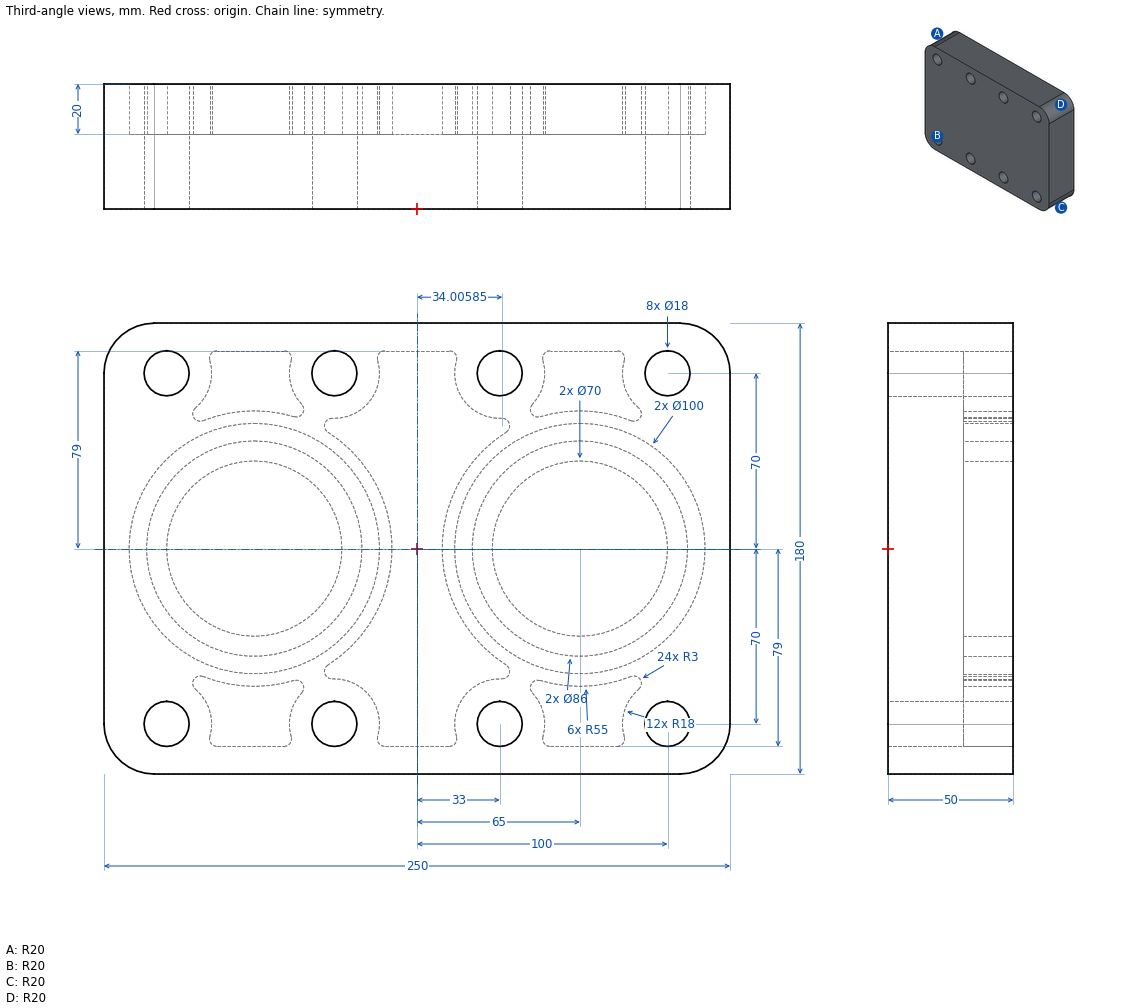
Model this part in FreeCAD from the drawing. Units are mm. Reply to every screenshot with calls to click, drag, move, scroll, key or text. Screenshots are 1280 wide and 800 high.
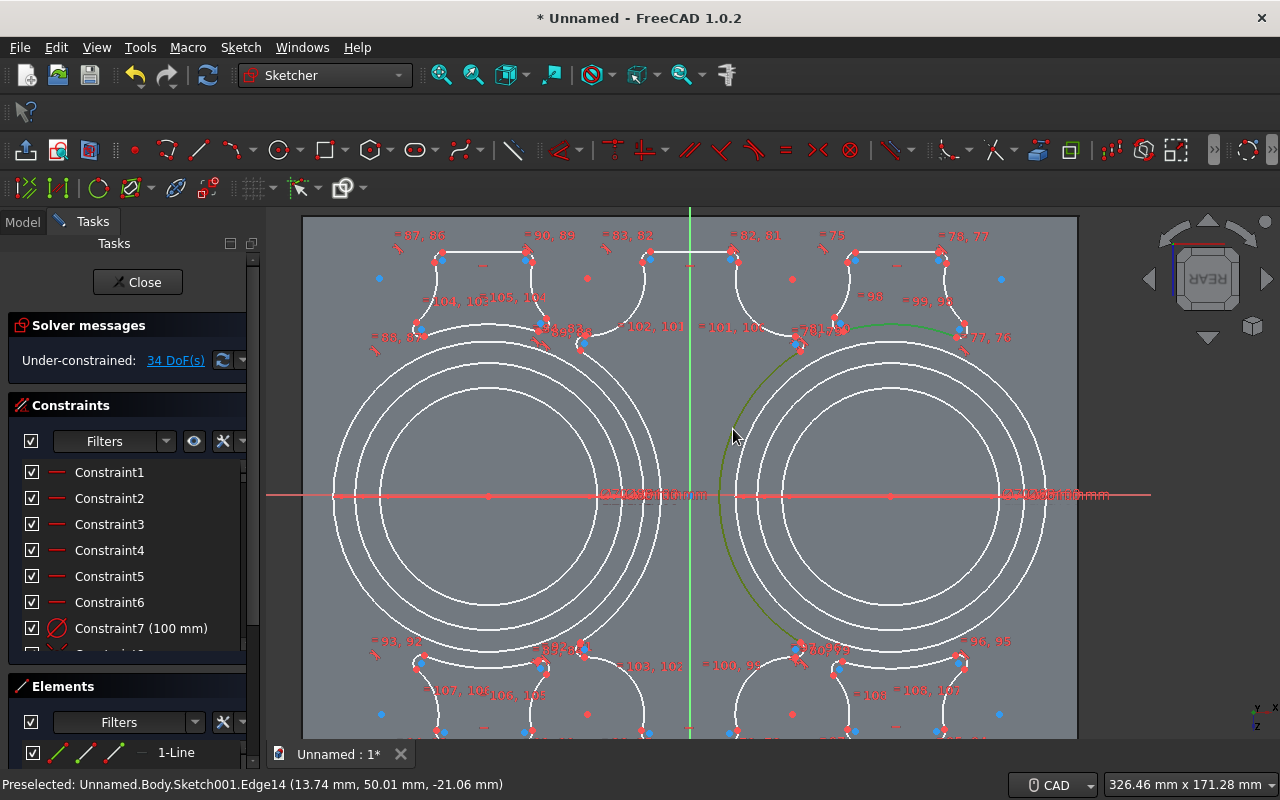
click(647, 564)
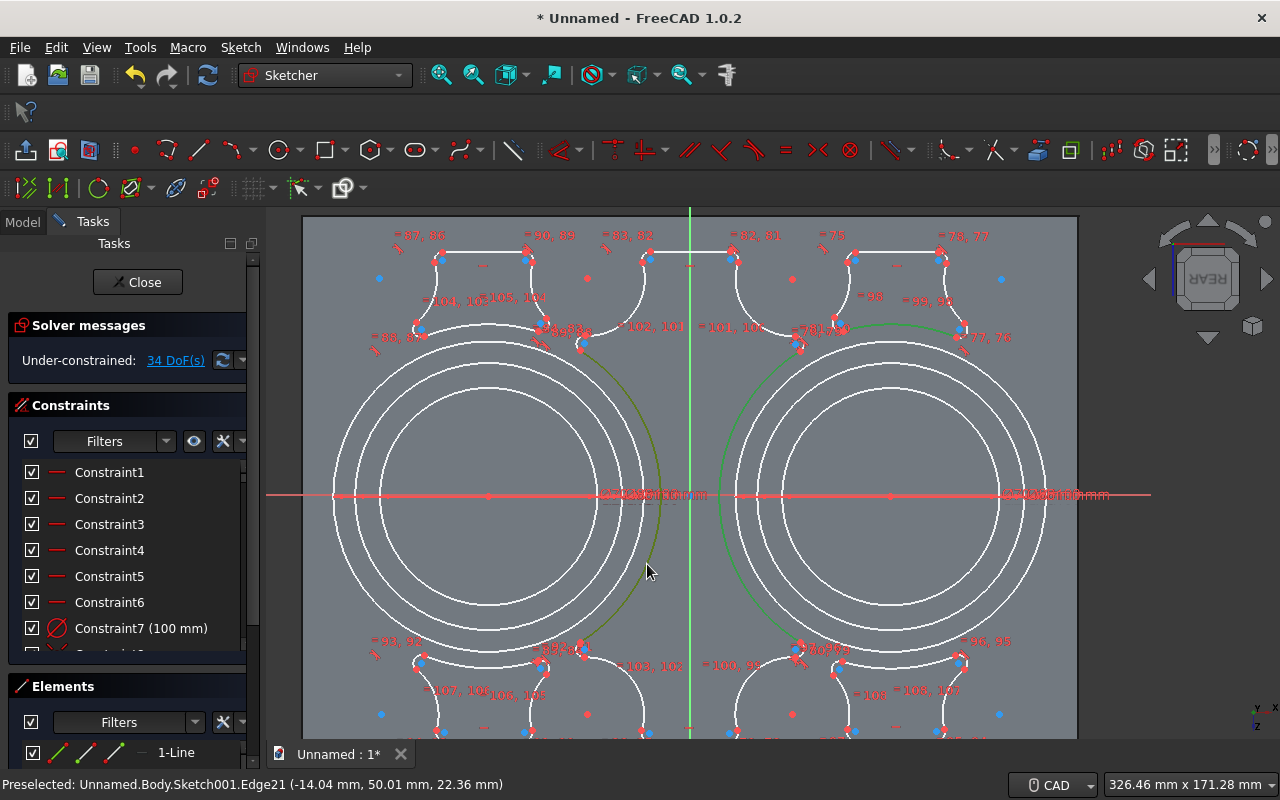
click(504, 325)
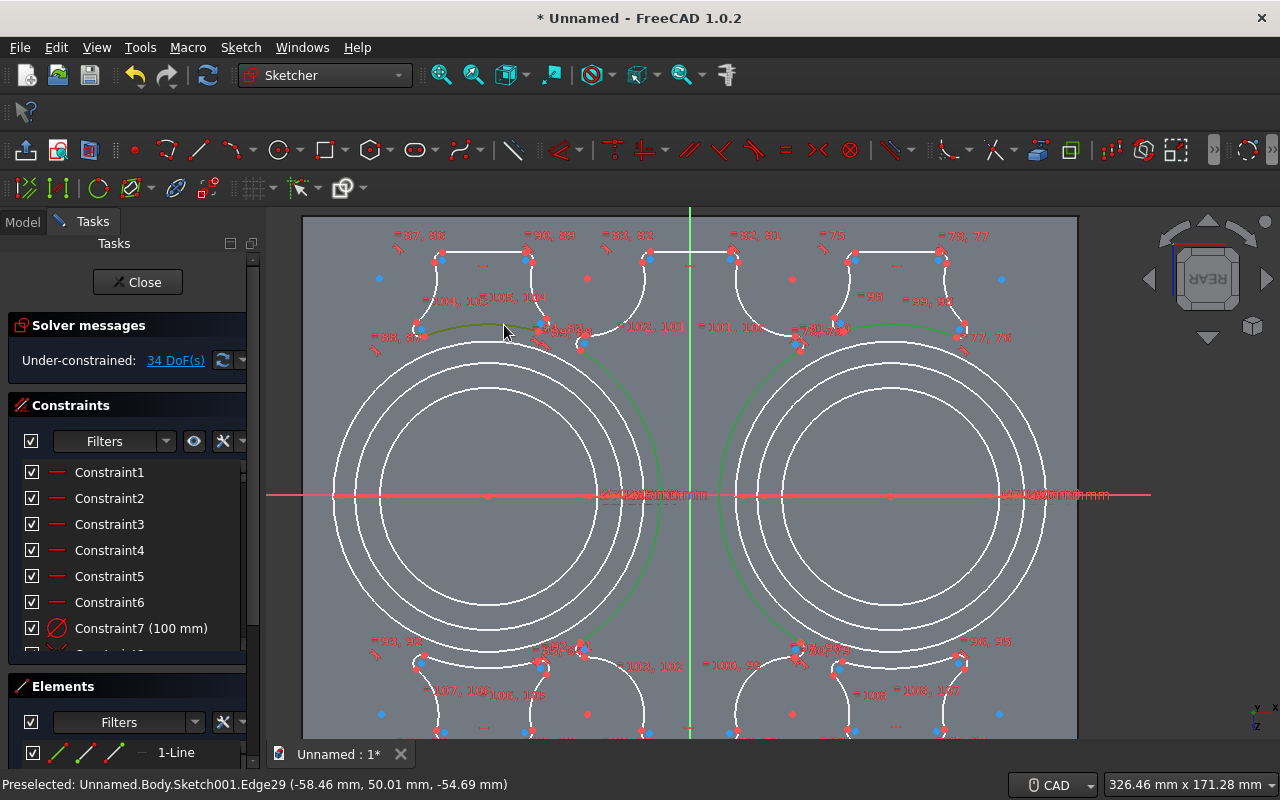
click(458, 665)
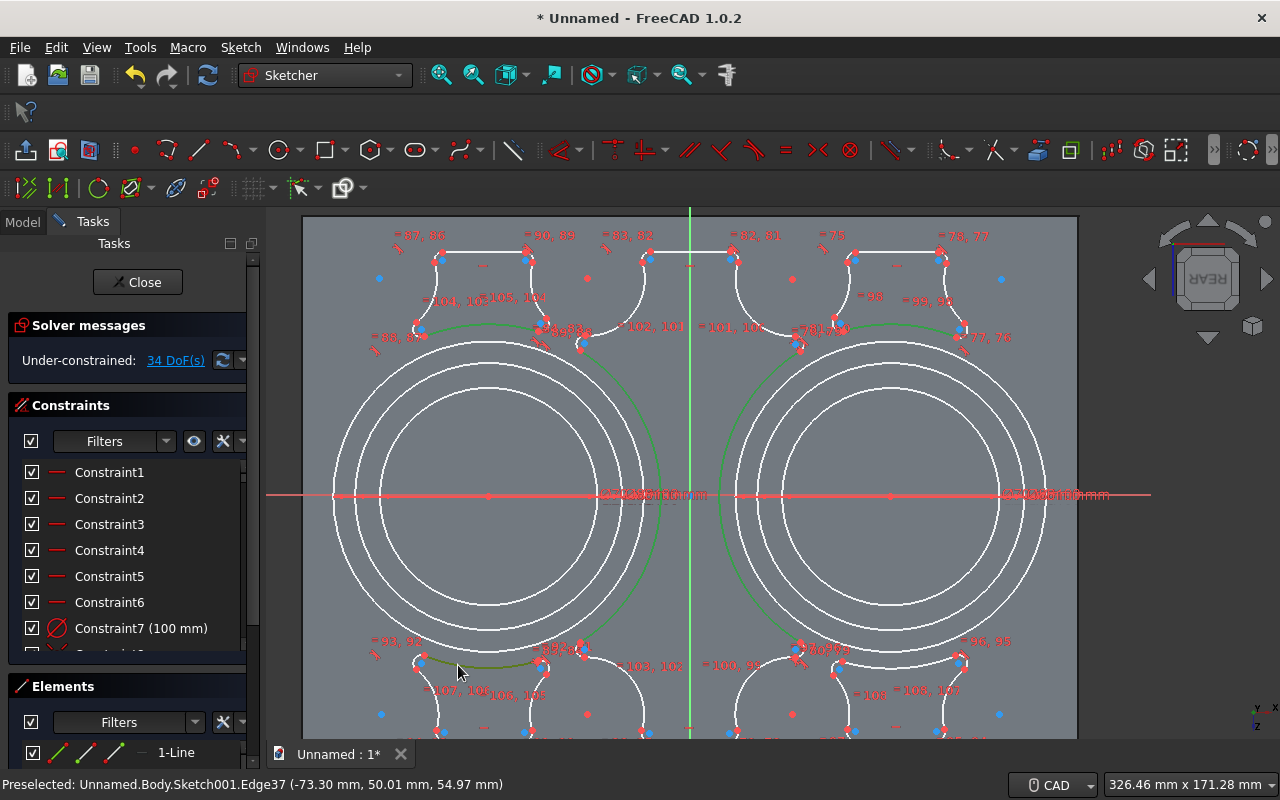
click(876, 668)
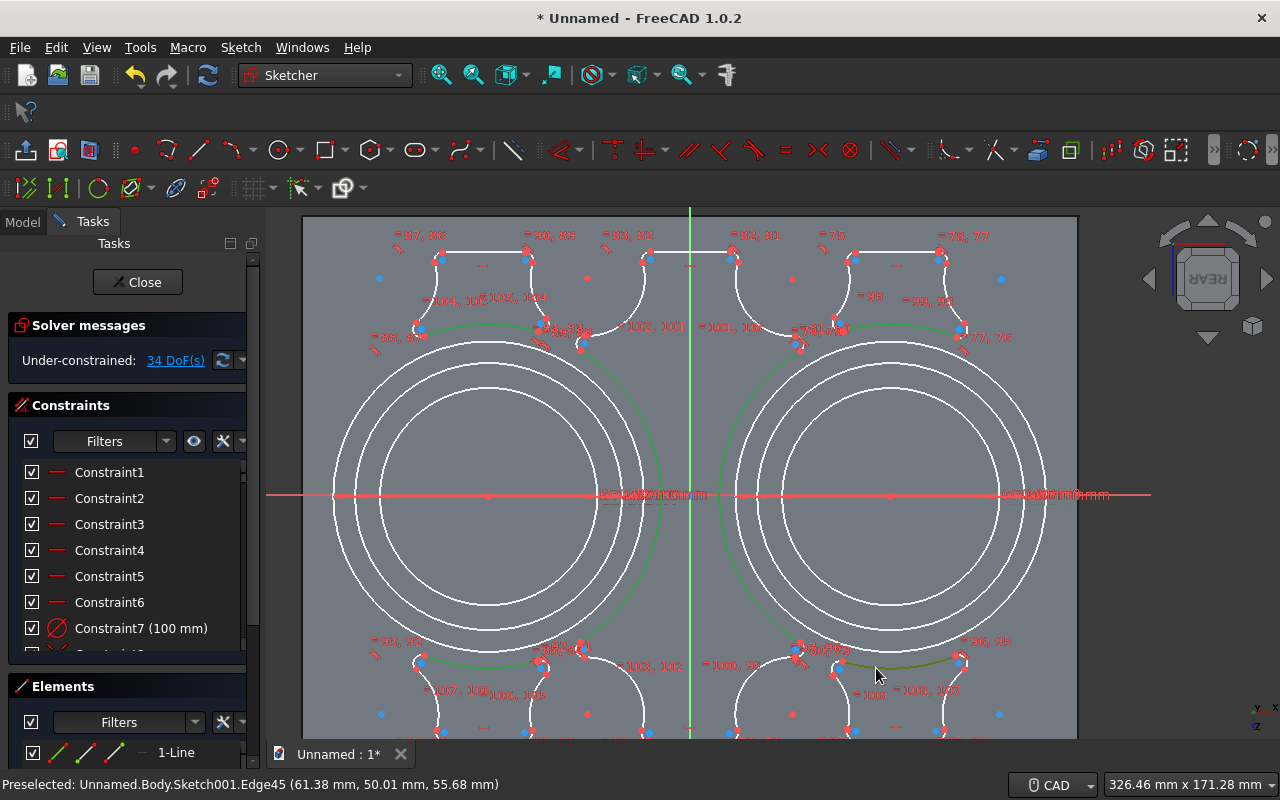
click(786, 150)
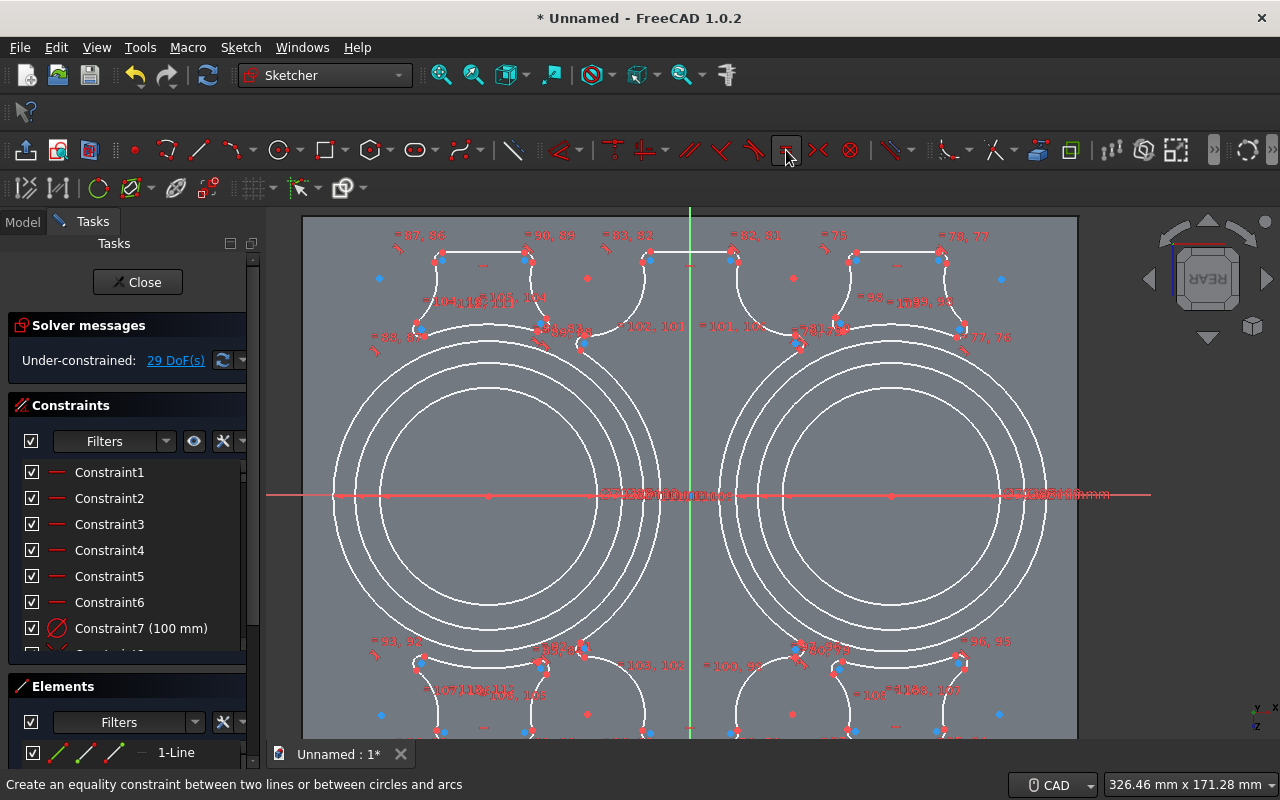
click(891, 496)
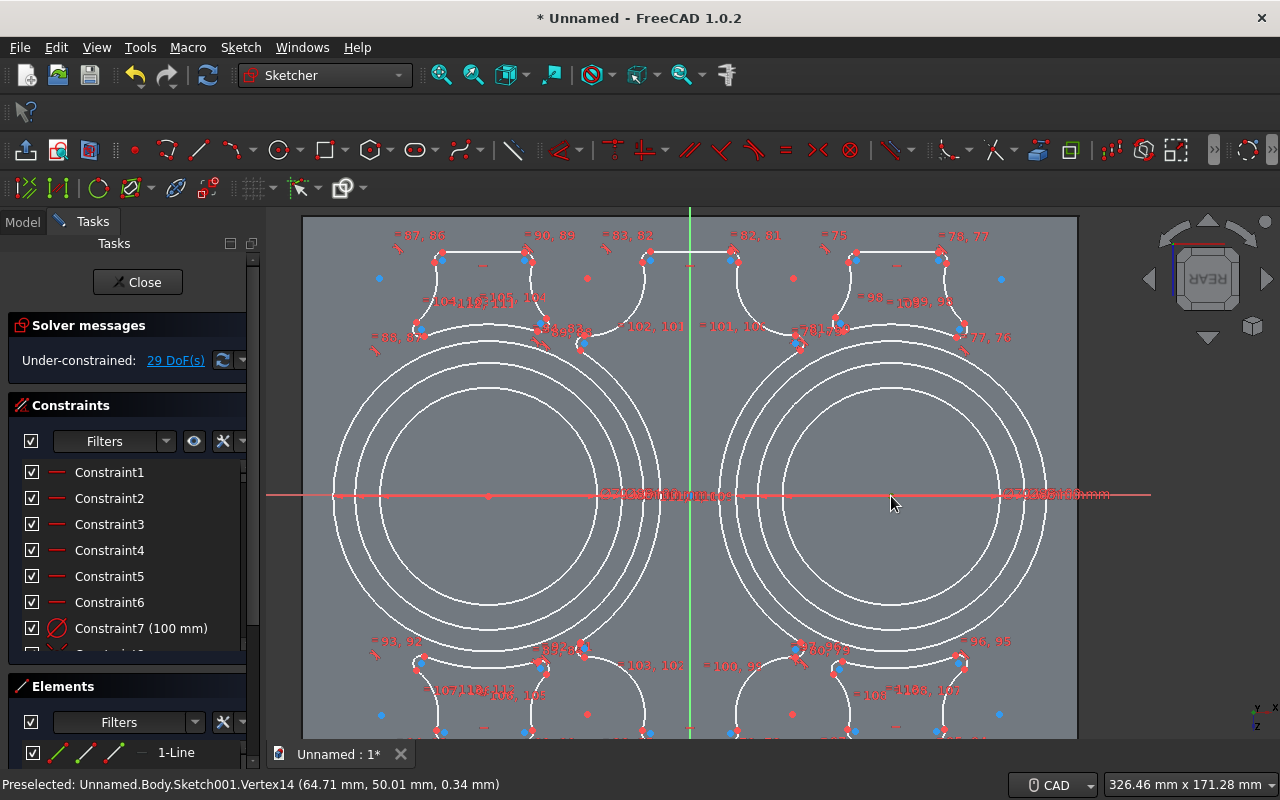
click(411, 495)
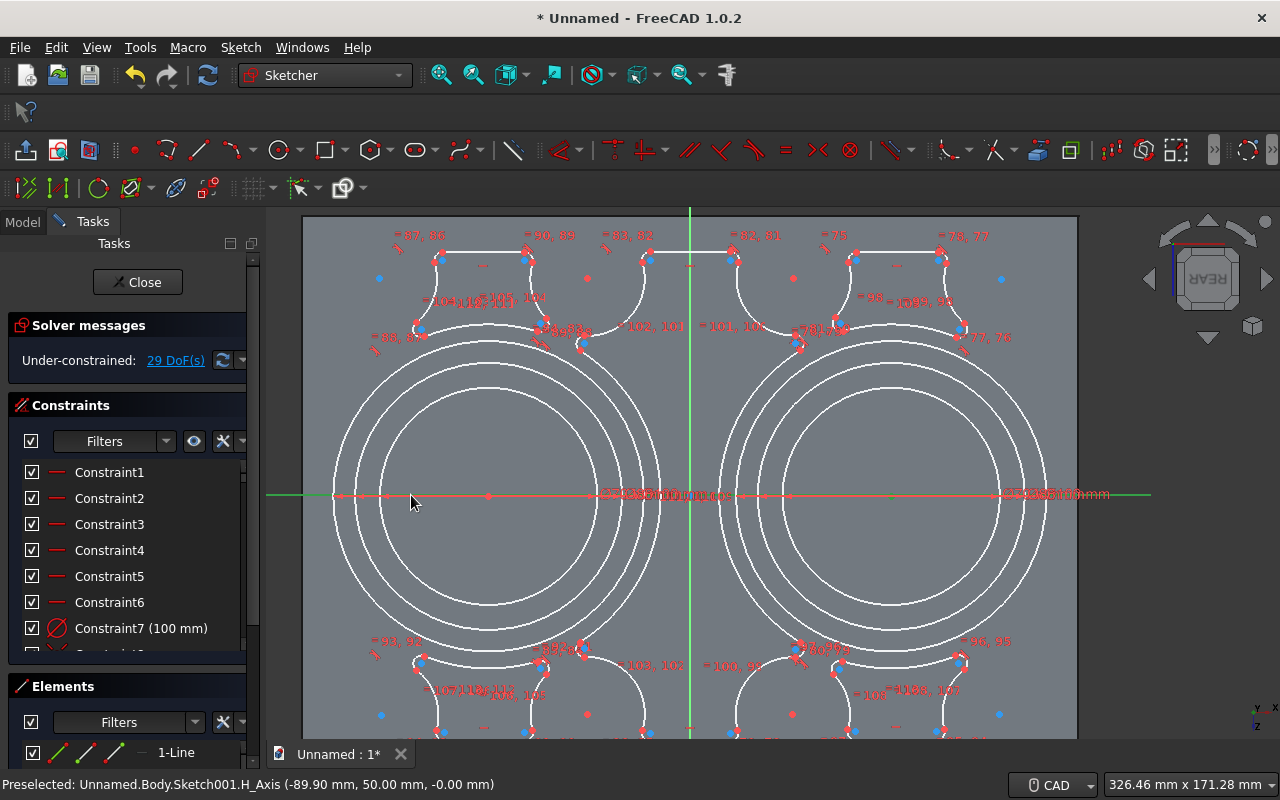
click(614, 150)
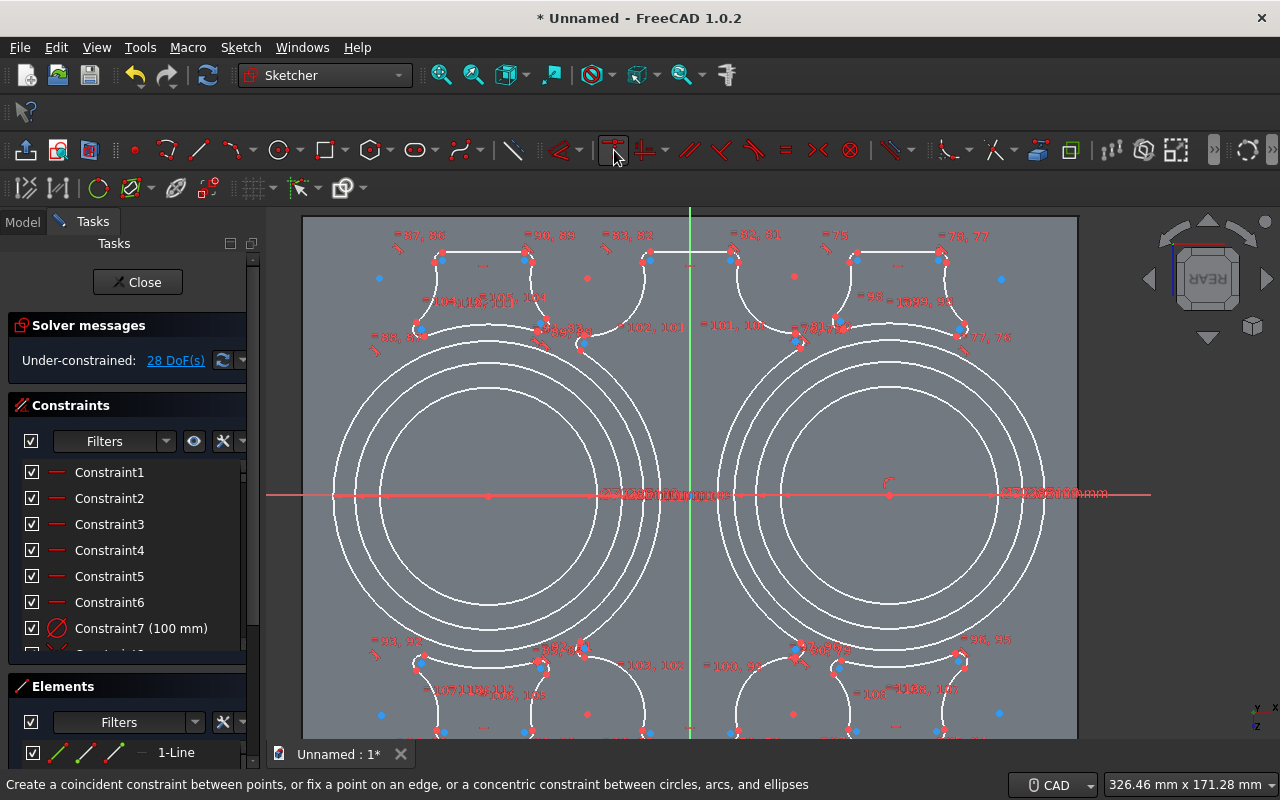
click(489, 496)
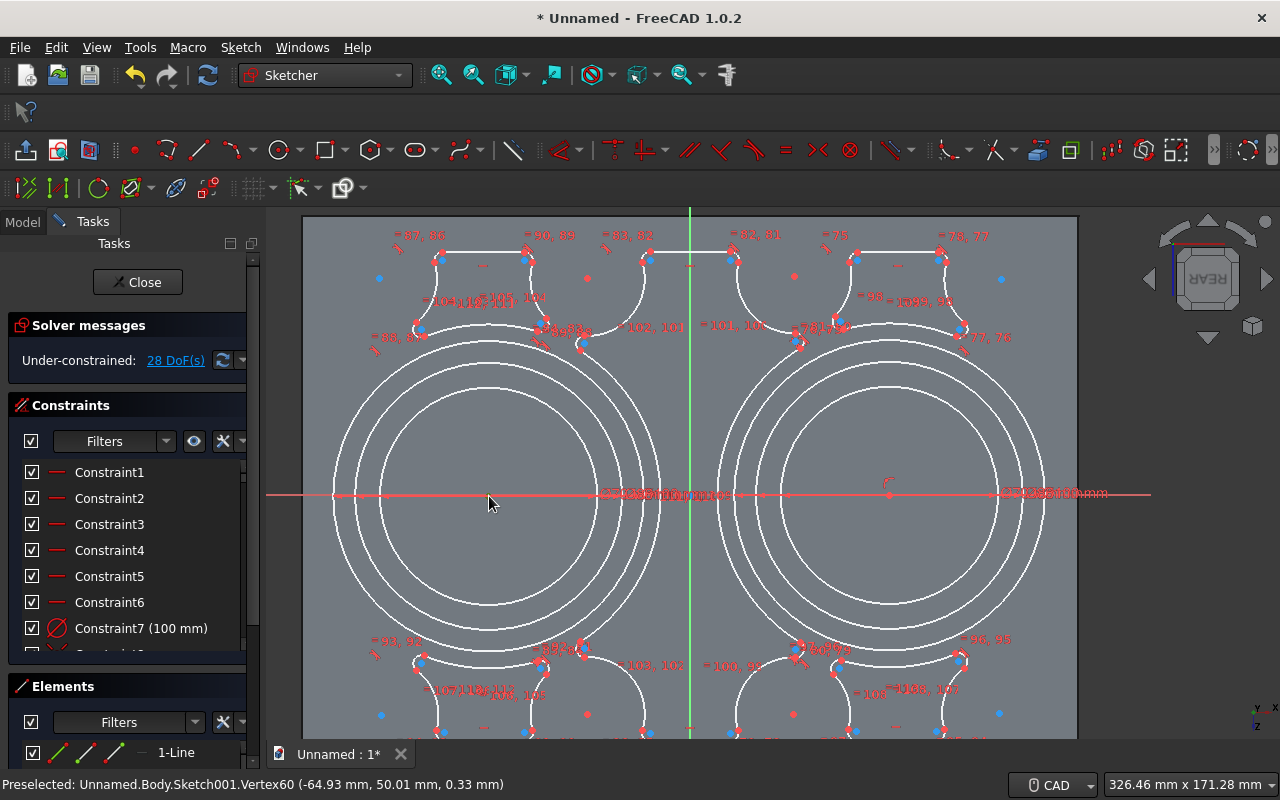
click(411, 495)